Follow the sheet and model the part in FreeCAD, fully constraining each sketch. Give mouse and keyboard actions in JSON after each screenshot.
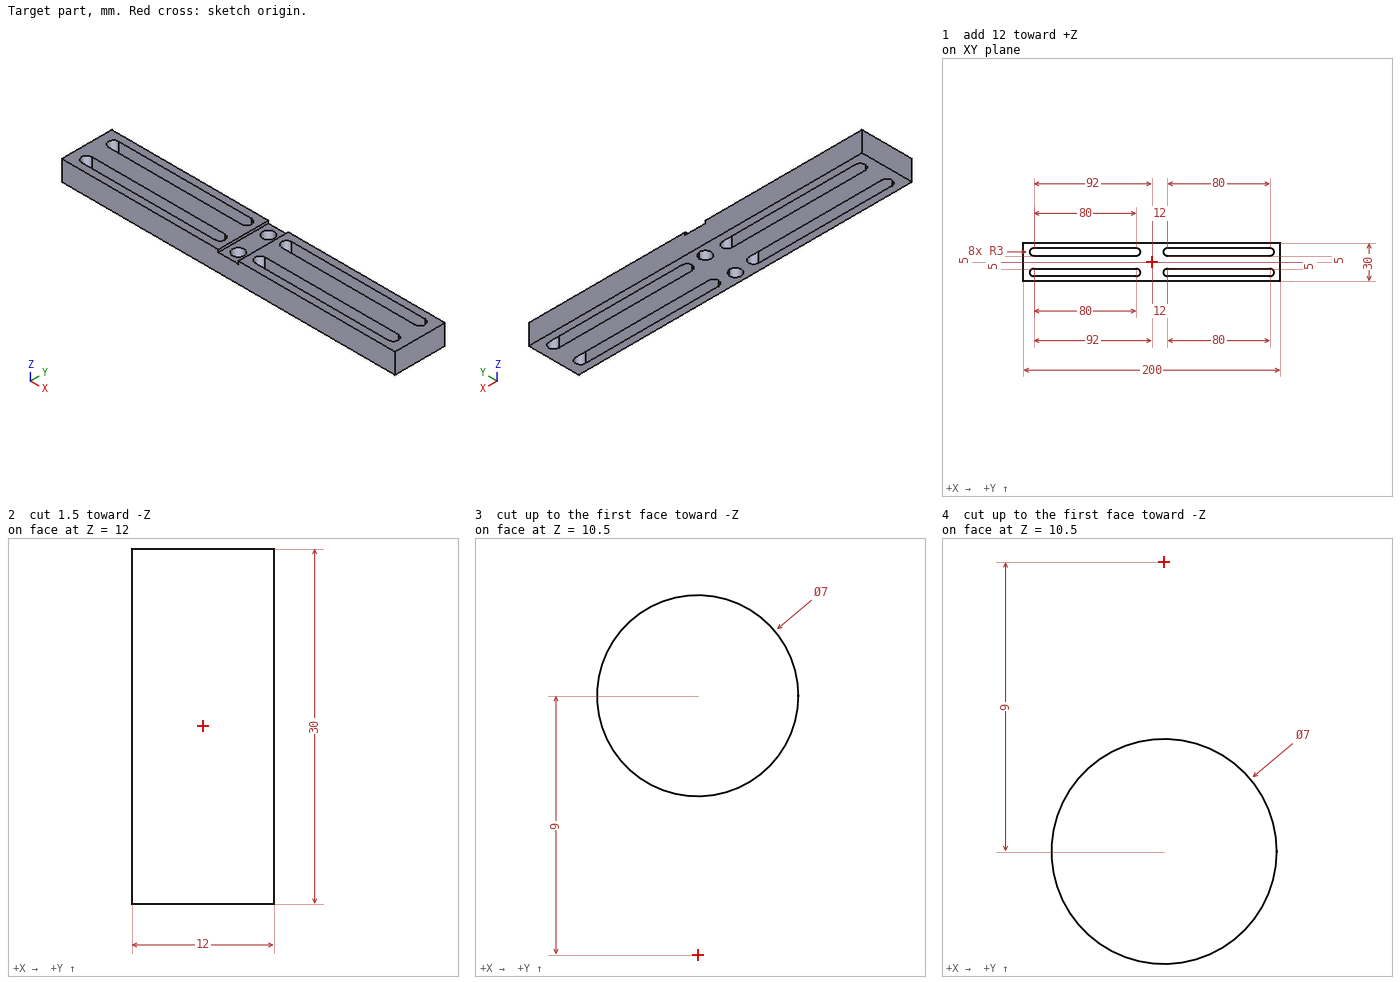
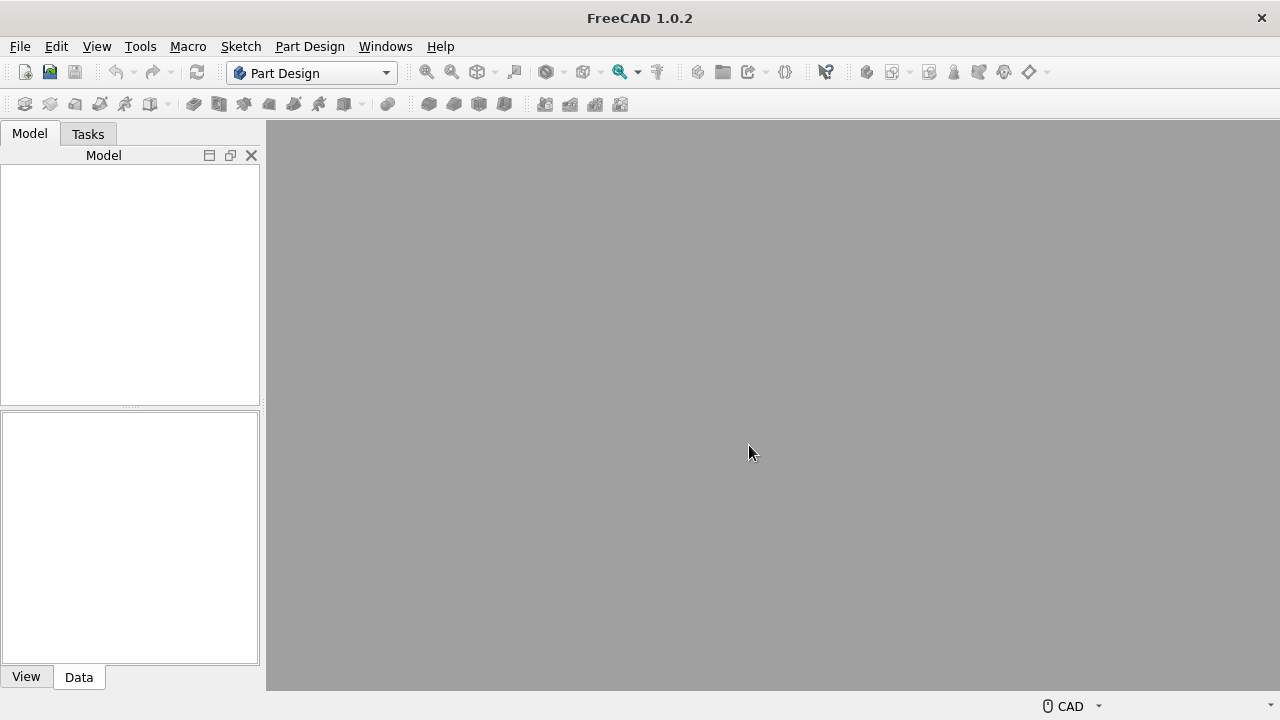
{"action": "left_click", "coordinate": [25, 72]}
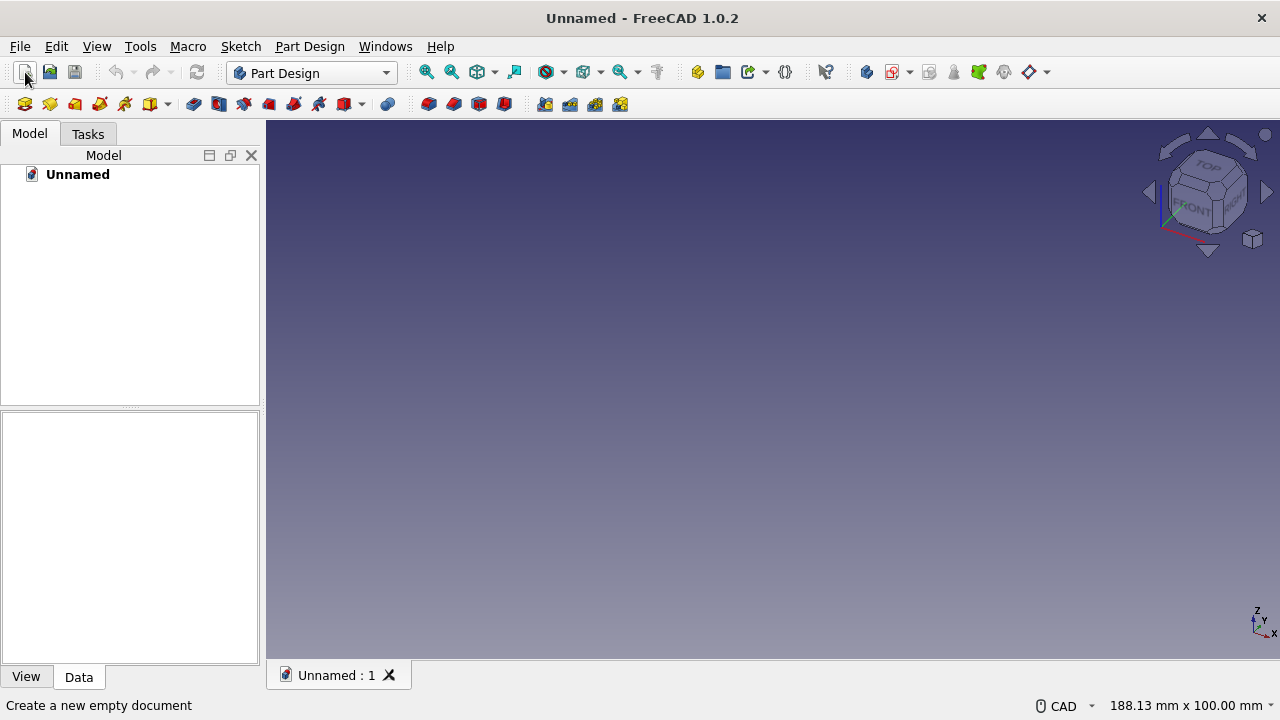
{"action": "left_click", "coordinate": [892, 72]}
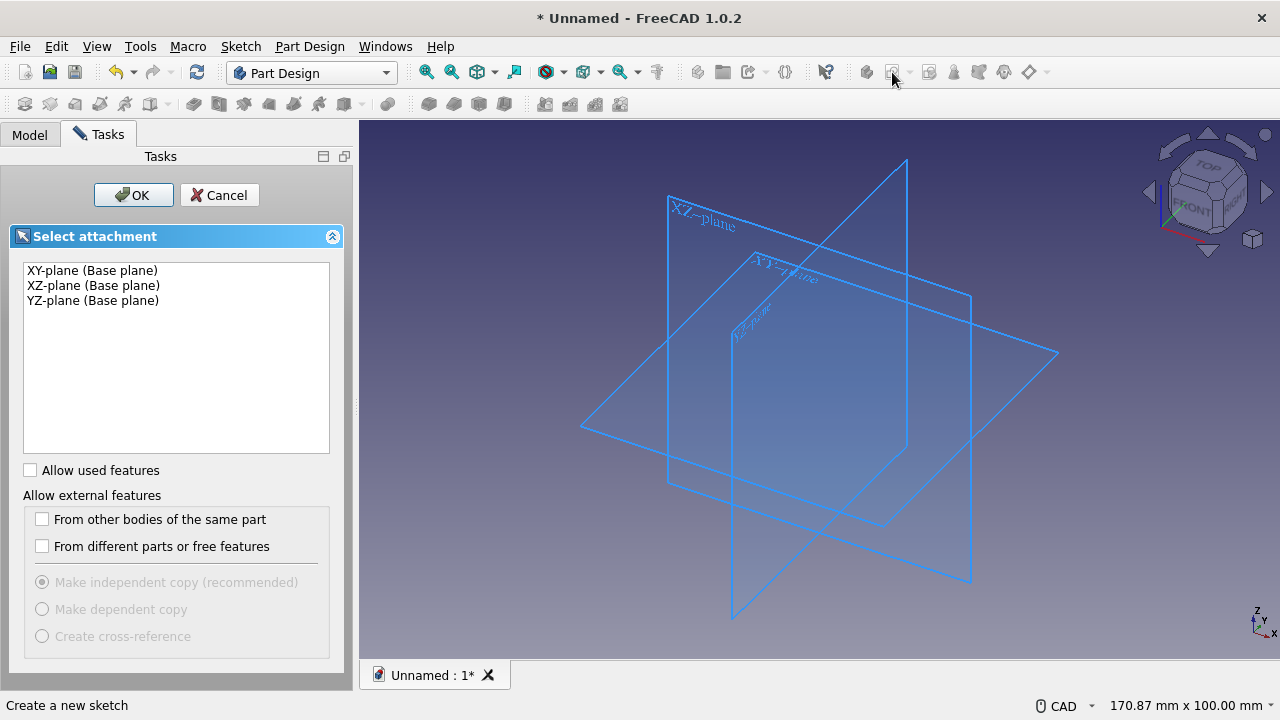
{"action": "left_click", "coordinate": [84, 270]}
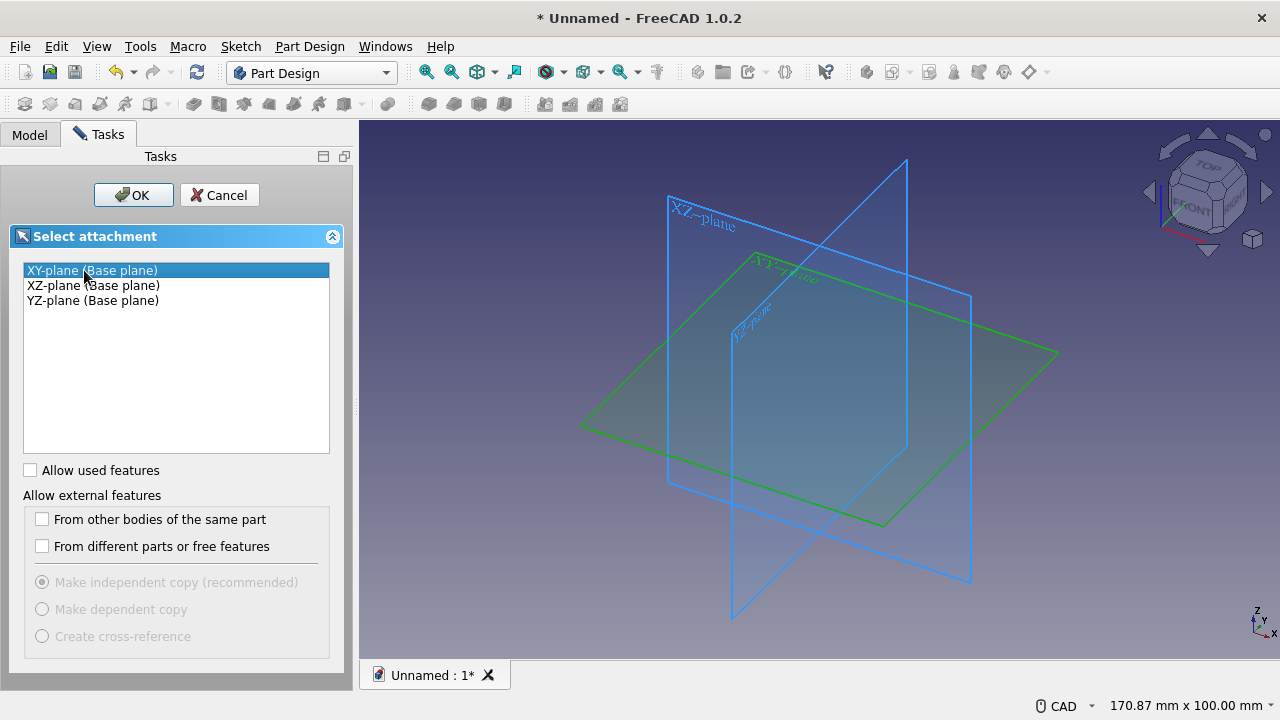
{"action": "left_click", "coordinate": [134, 195]}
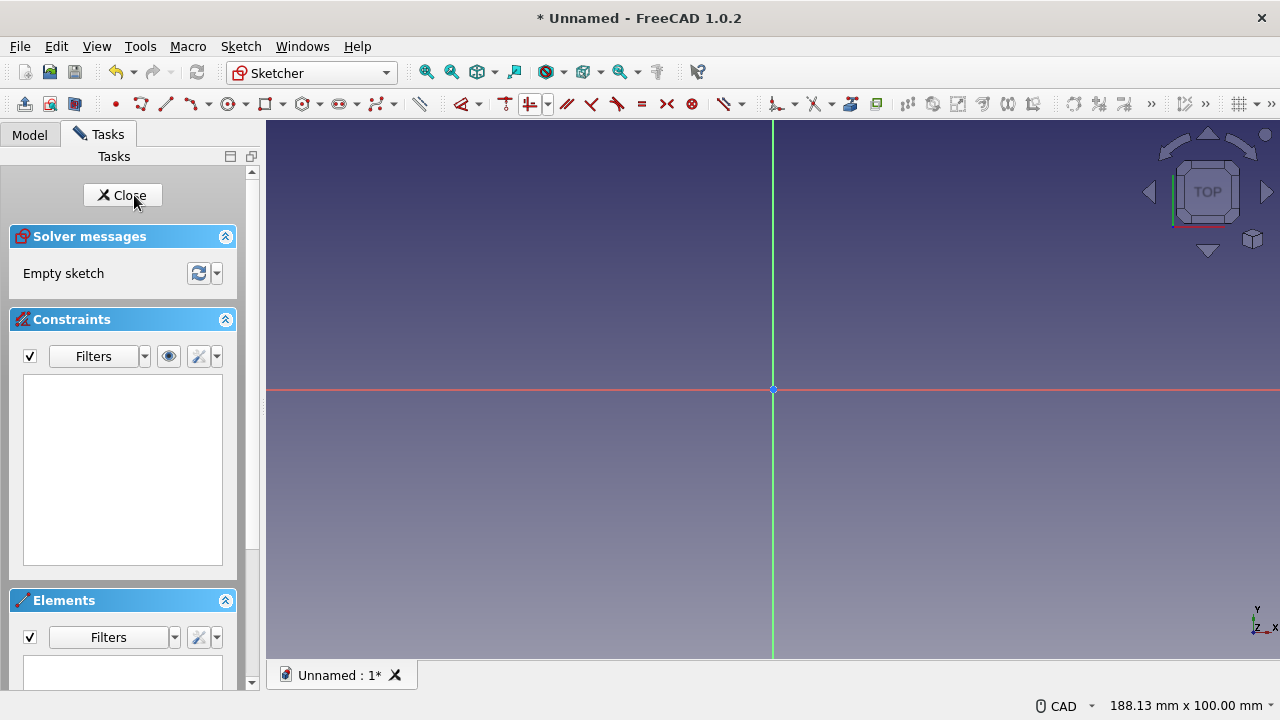
{"action": "scroll", "coordinate": [621, 390], "scroll_direction": "down", "scroll_amount": 3}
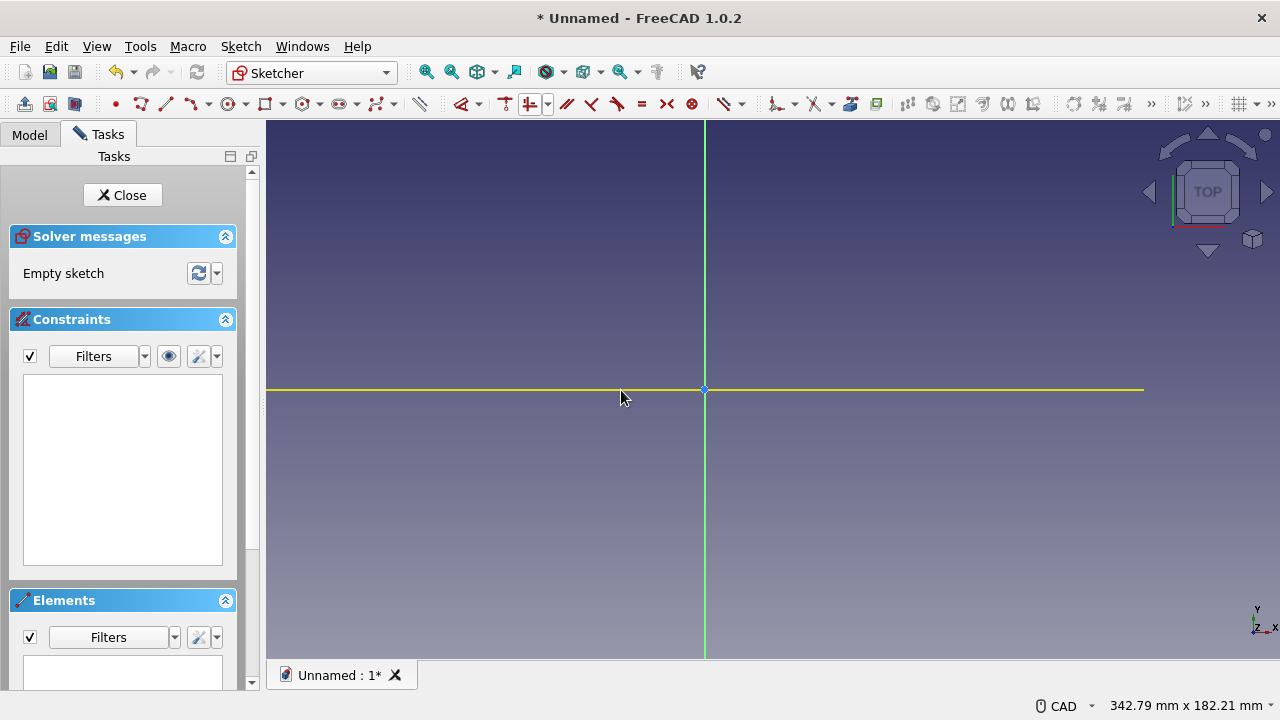
{"action": "left_click", "coordinate": [282, 104]}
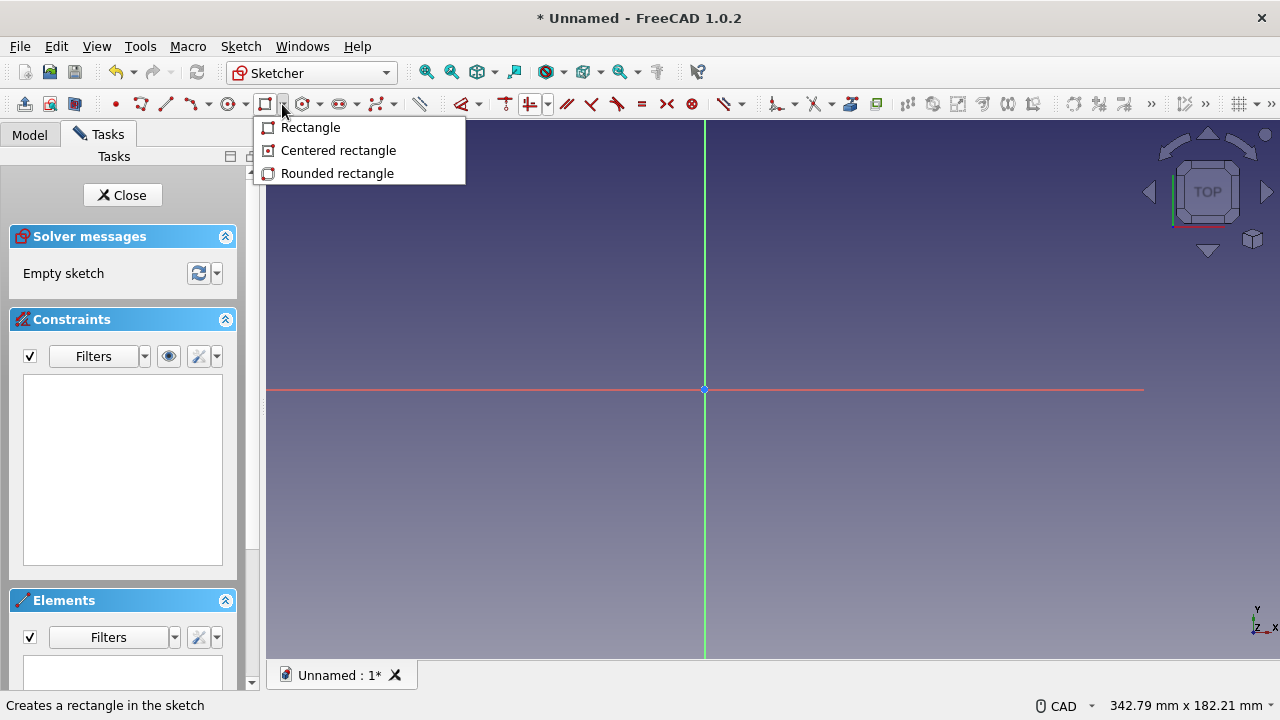
{"action": "left_click", "coordinate": [360, 150]}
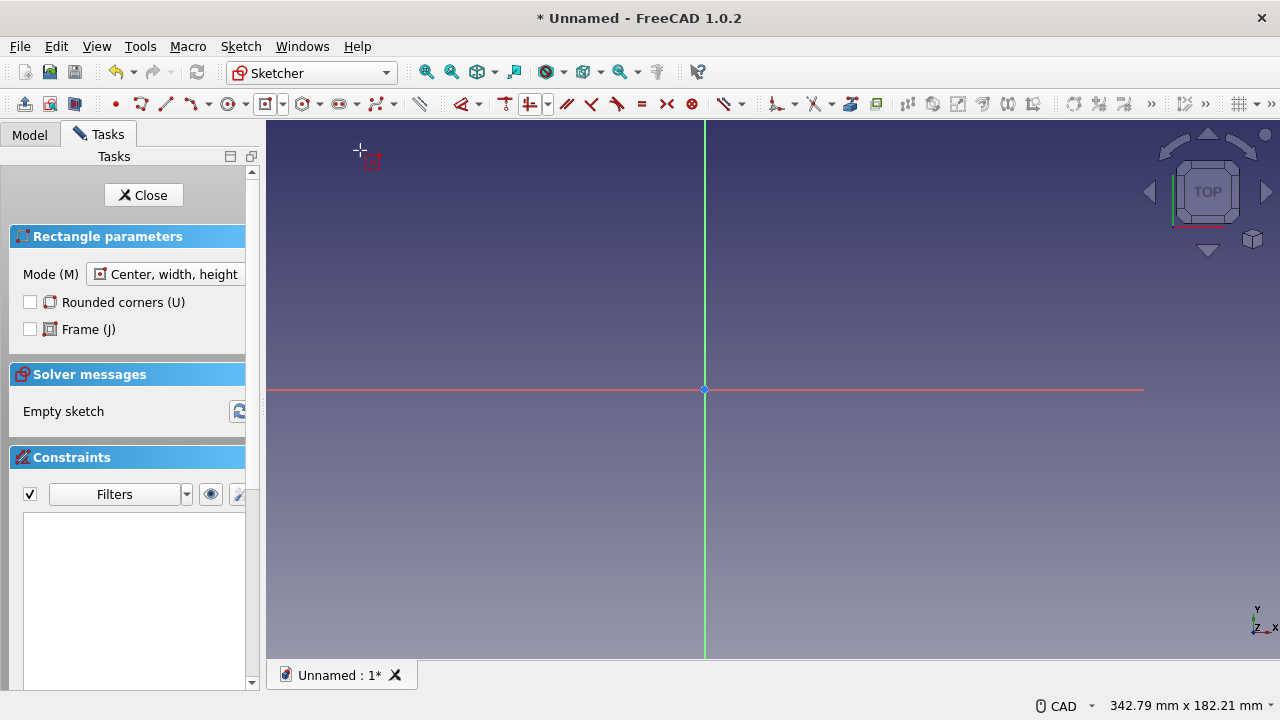
{"action": "left_click", "coordinate": [705, 390]}
{"action": "mouse_move", "coordinate": [1000, 346]}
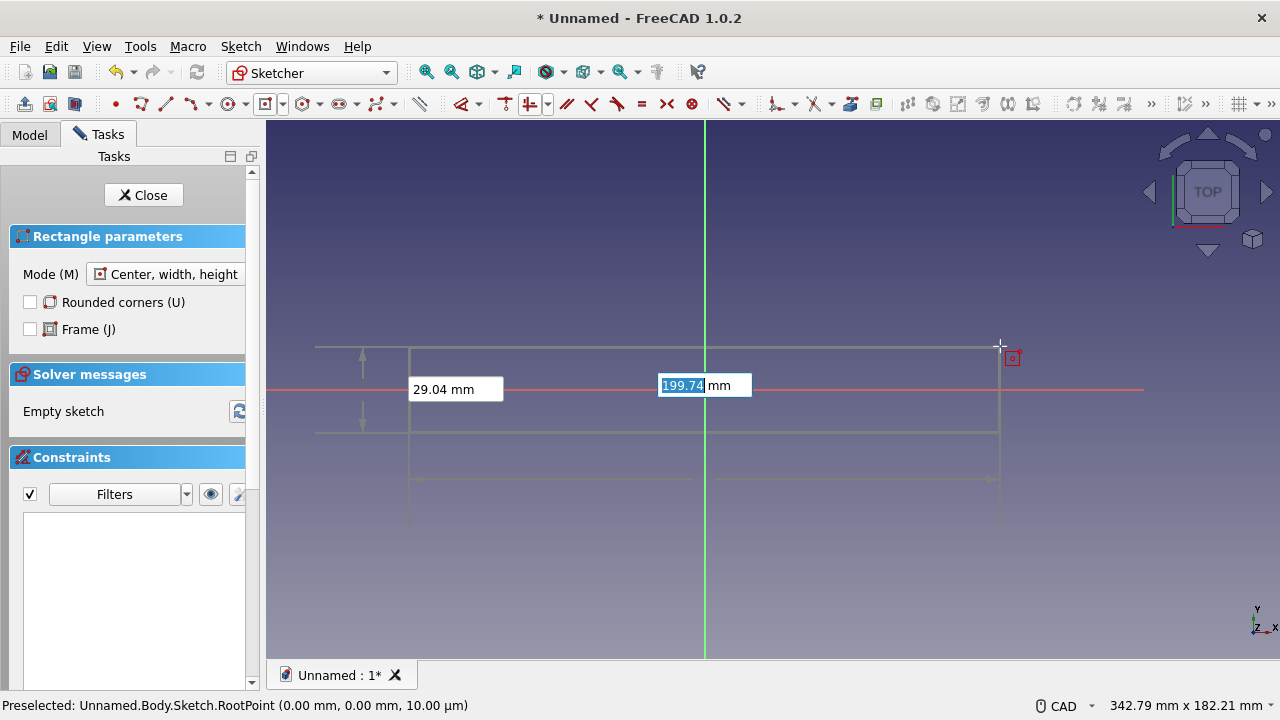
{"action": "type", "text": "200"}
{"action": "key", "text": "Tab"}
{"action": "type", "text": "30"}
{"action": "key", "text": "Return"}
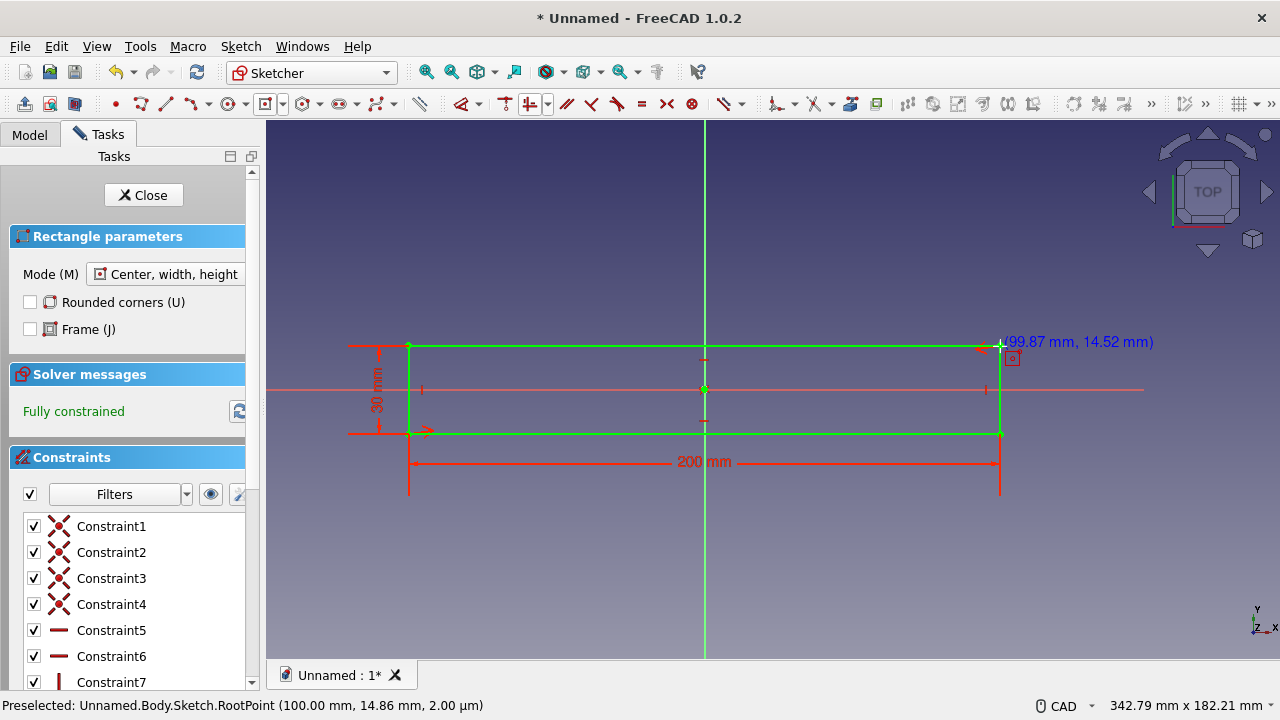
{"action": "left_click", "coordinate": [338, 104]}